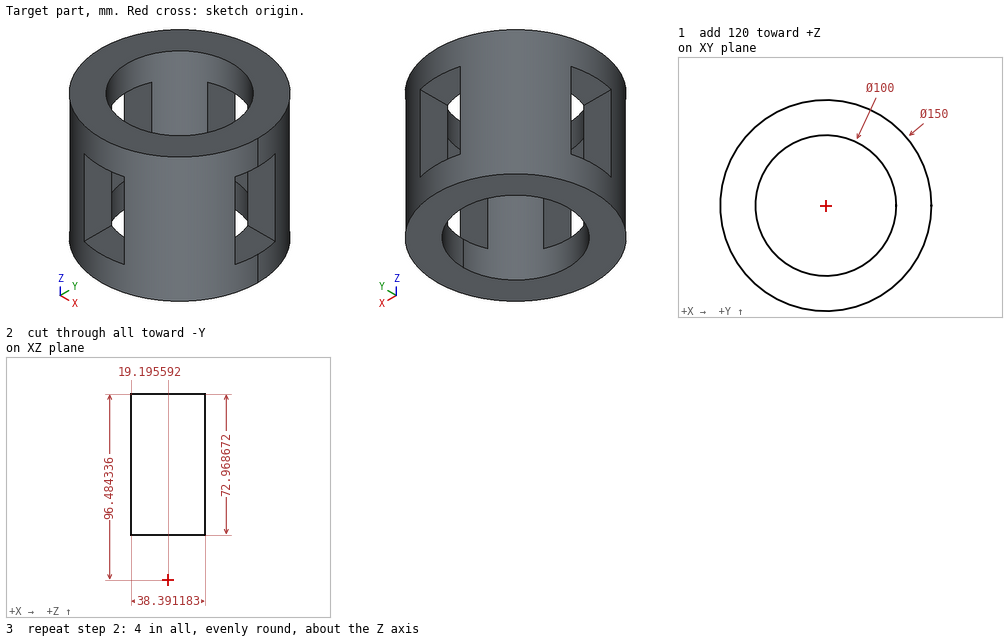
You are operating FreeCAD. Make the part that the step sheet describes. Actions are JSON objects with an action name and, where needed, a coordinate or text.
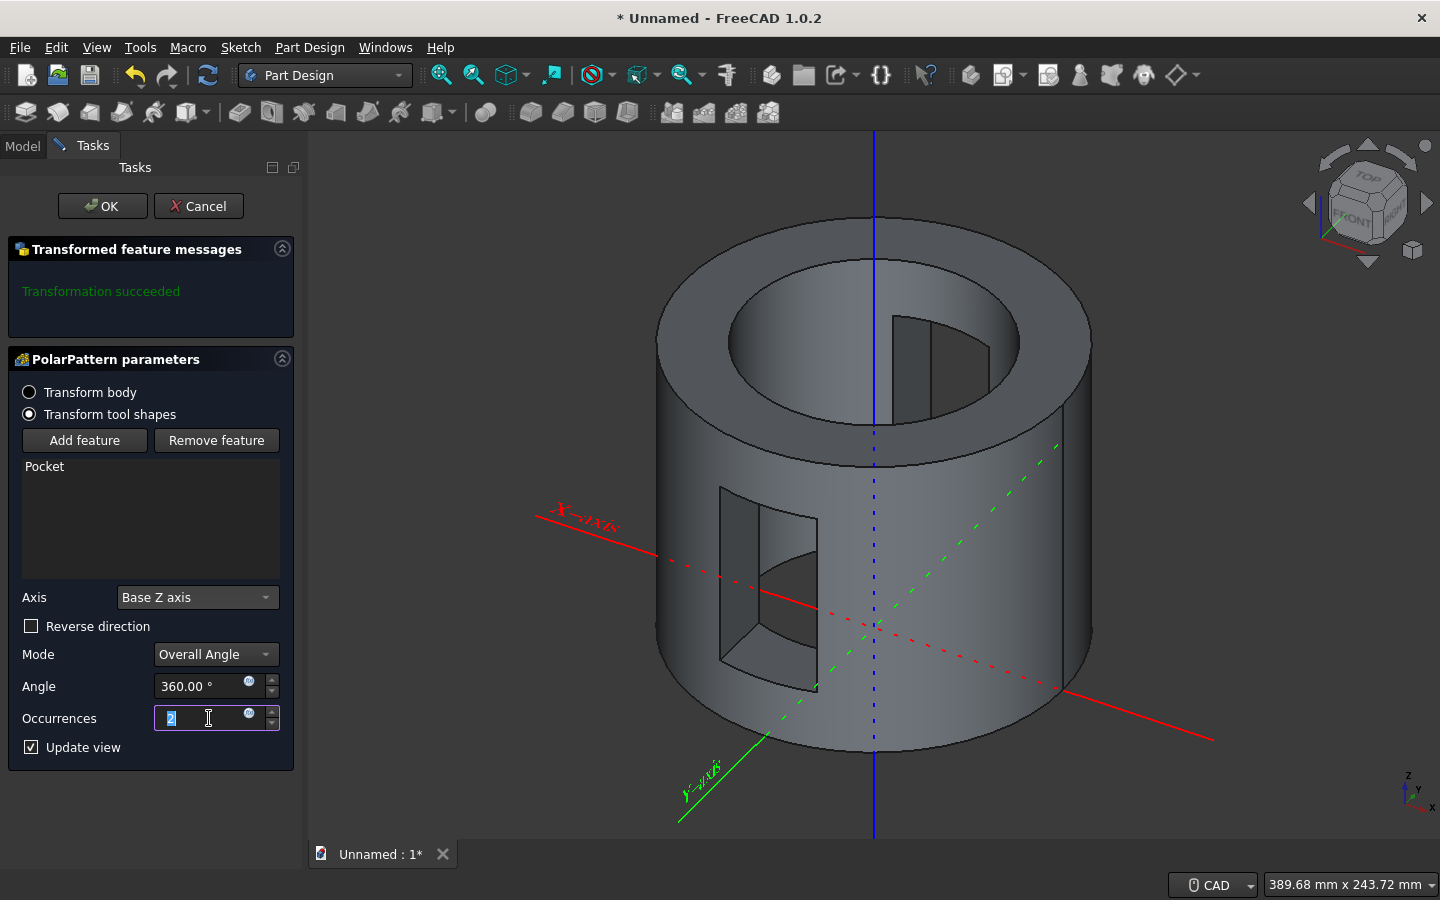
{"action": "type", "text": "4"}
{"action": "key", "text": "Tab"}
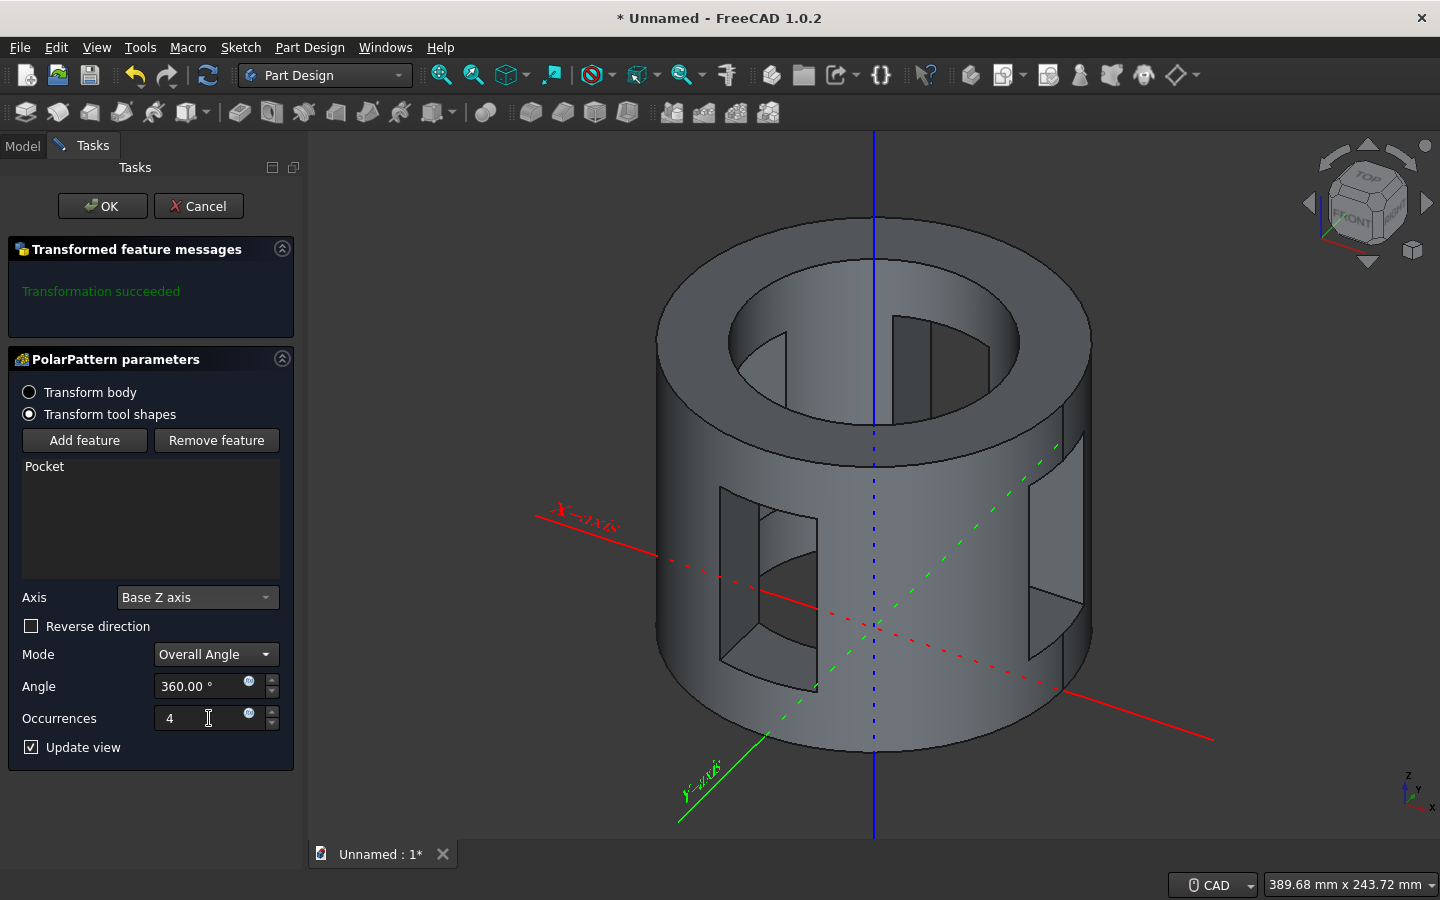
{"action": "left_click", "coordinate": [103, 206]}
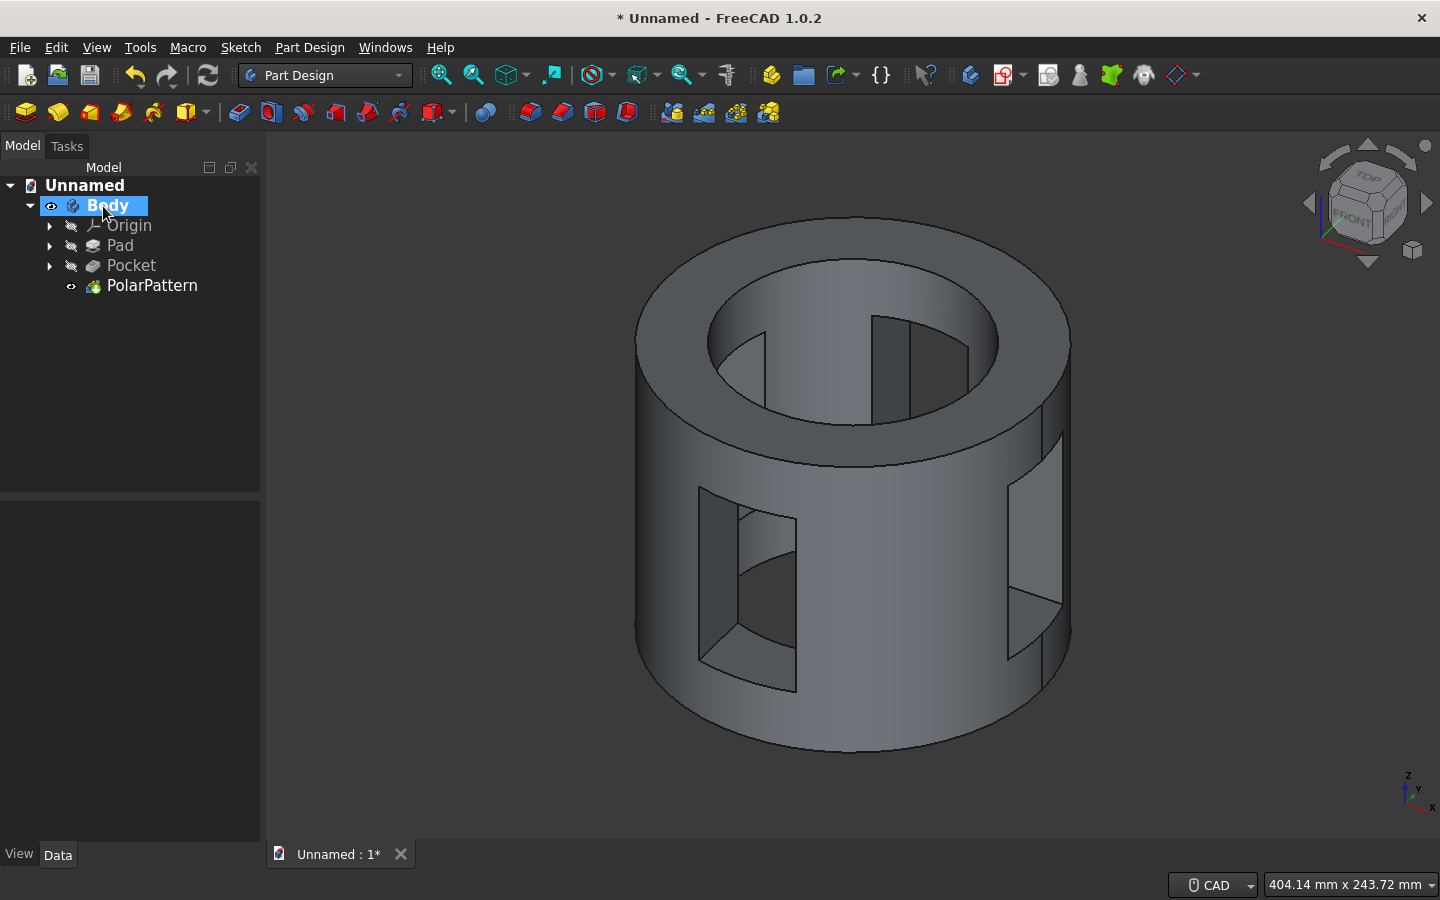
{"action": "key", "text": "0"}